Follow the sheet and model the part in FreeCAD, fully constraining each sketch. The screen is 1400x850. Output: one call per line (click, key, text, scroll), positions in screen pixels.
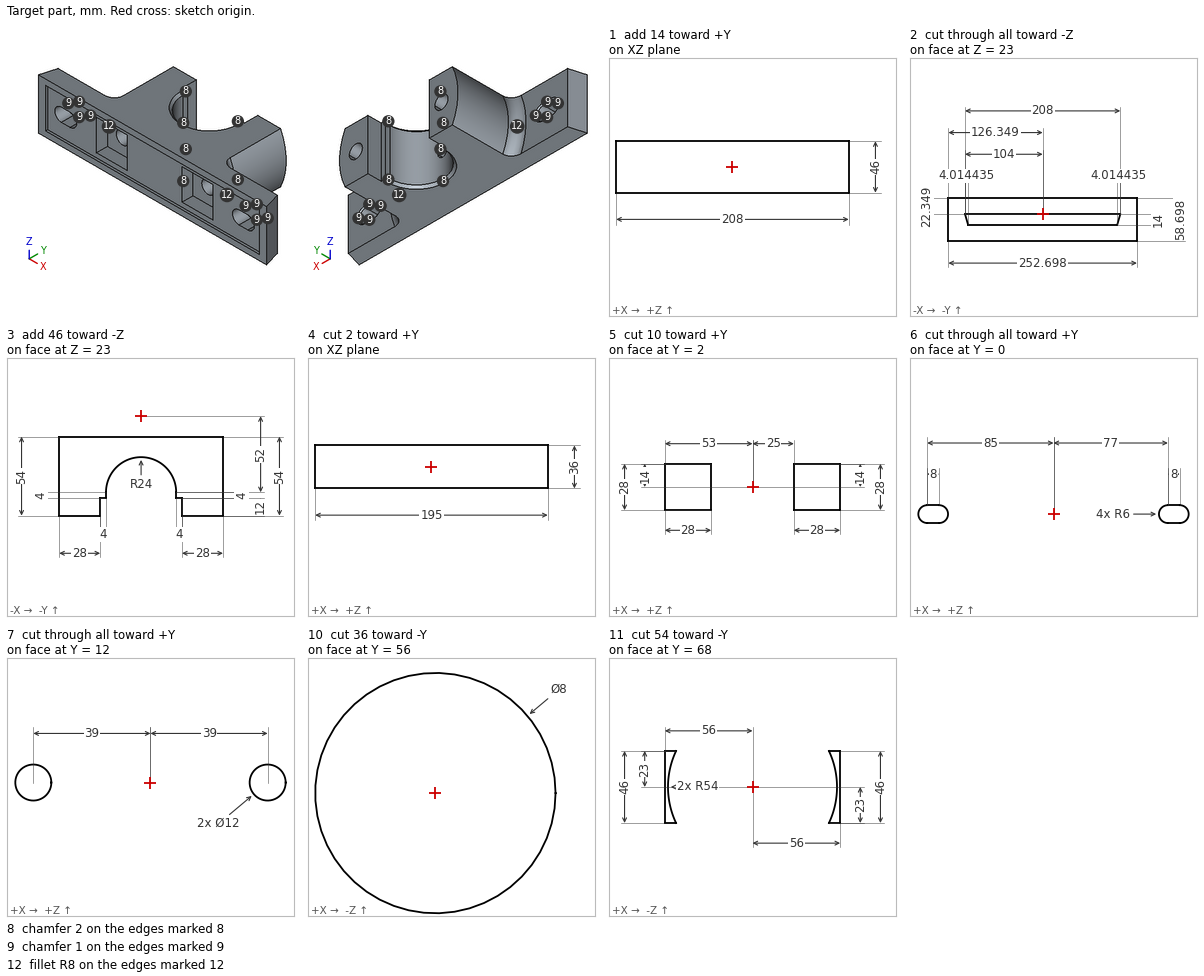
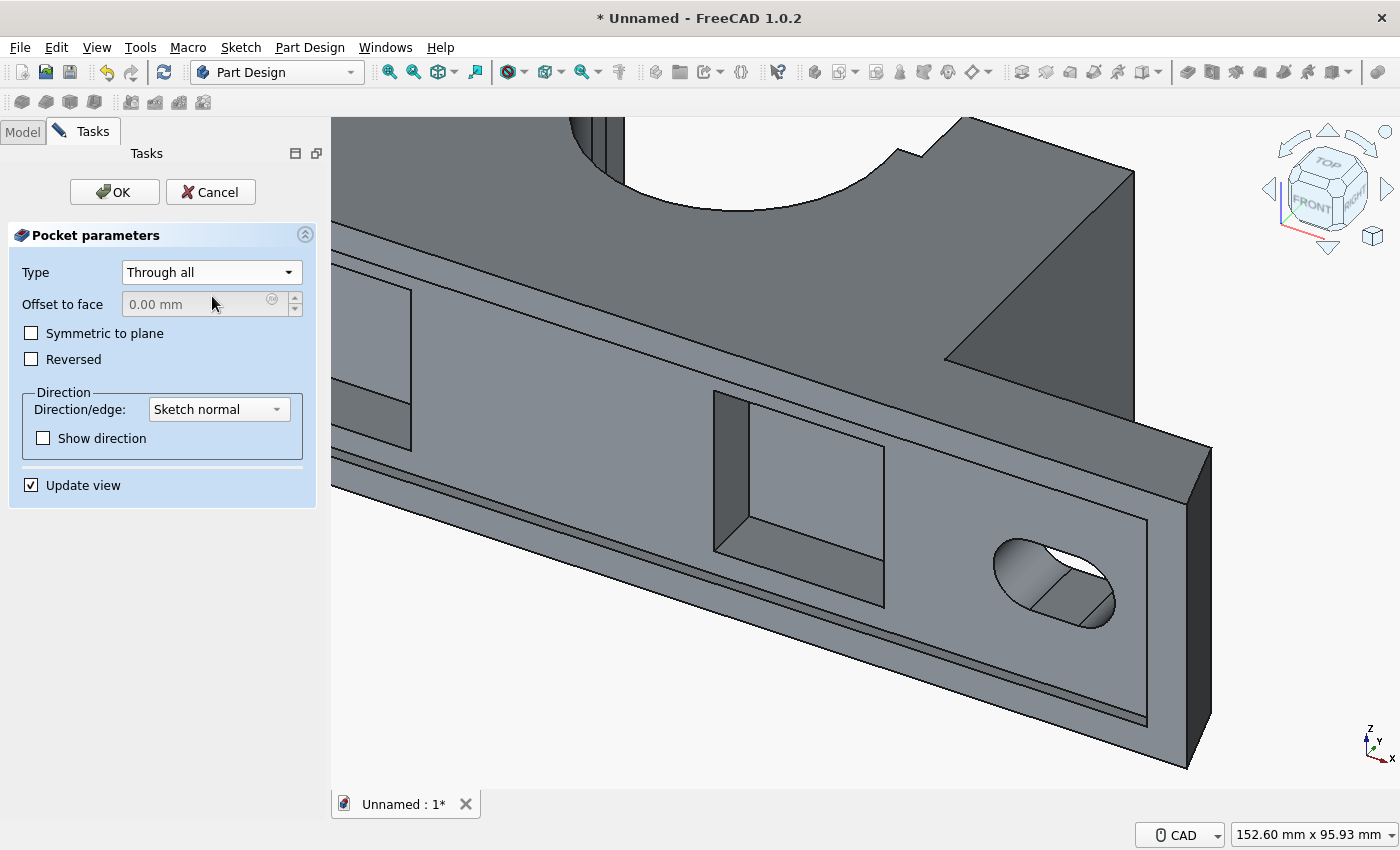
click(115, 192)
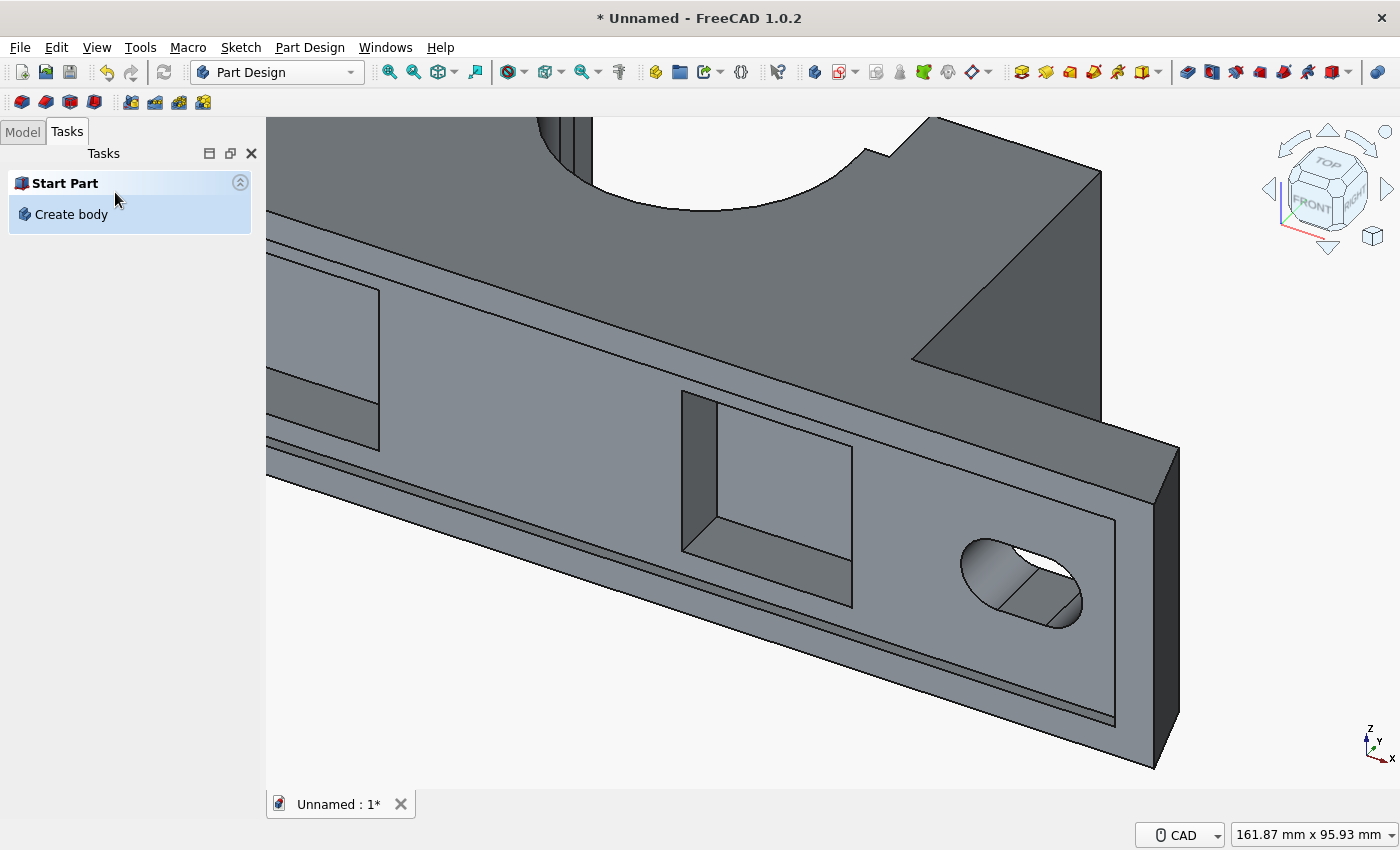
click(390, 72)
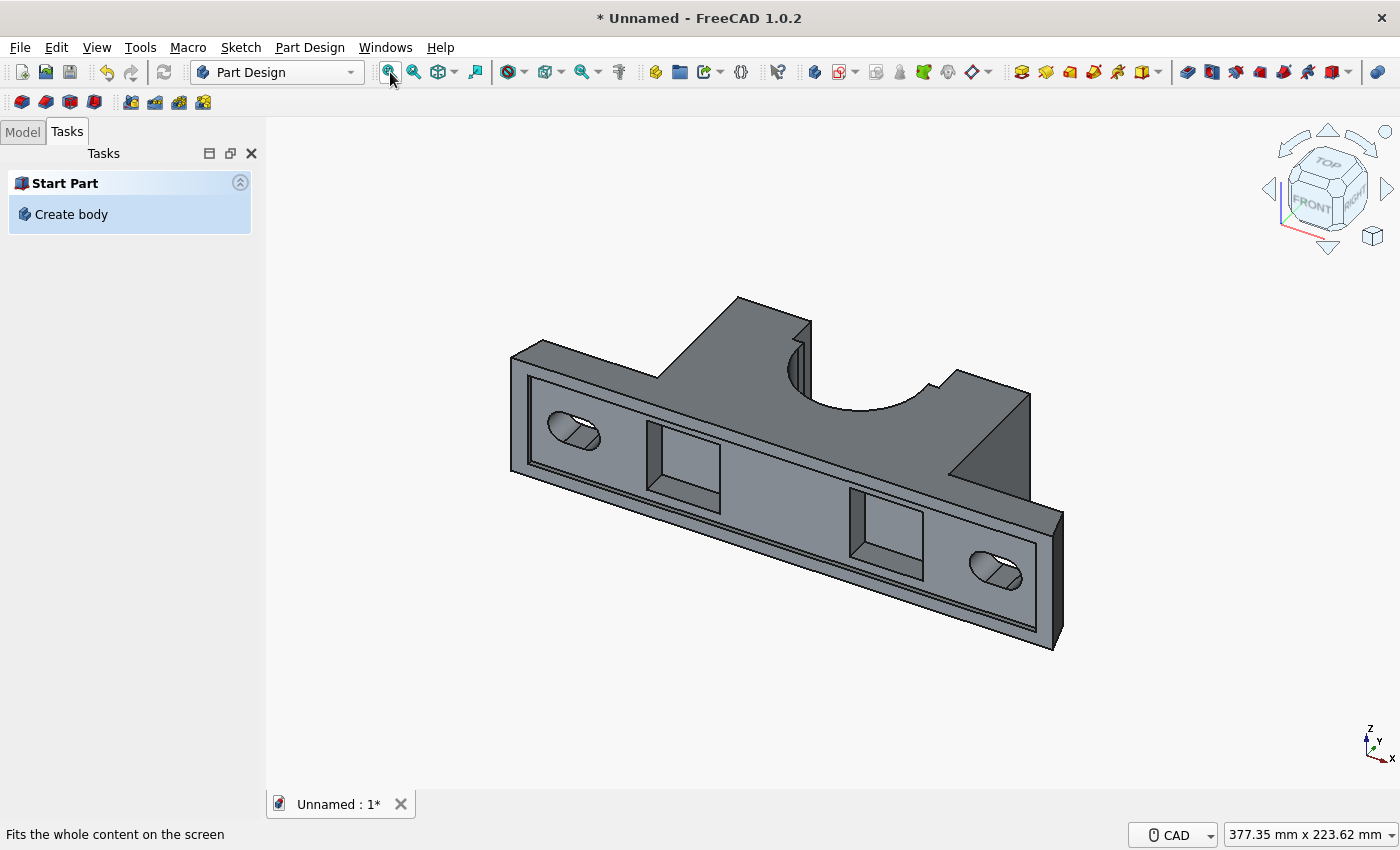
click(901, 518)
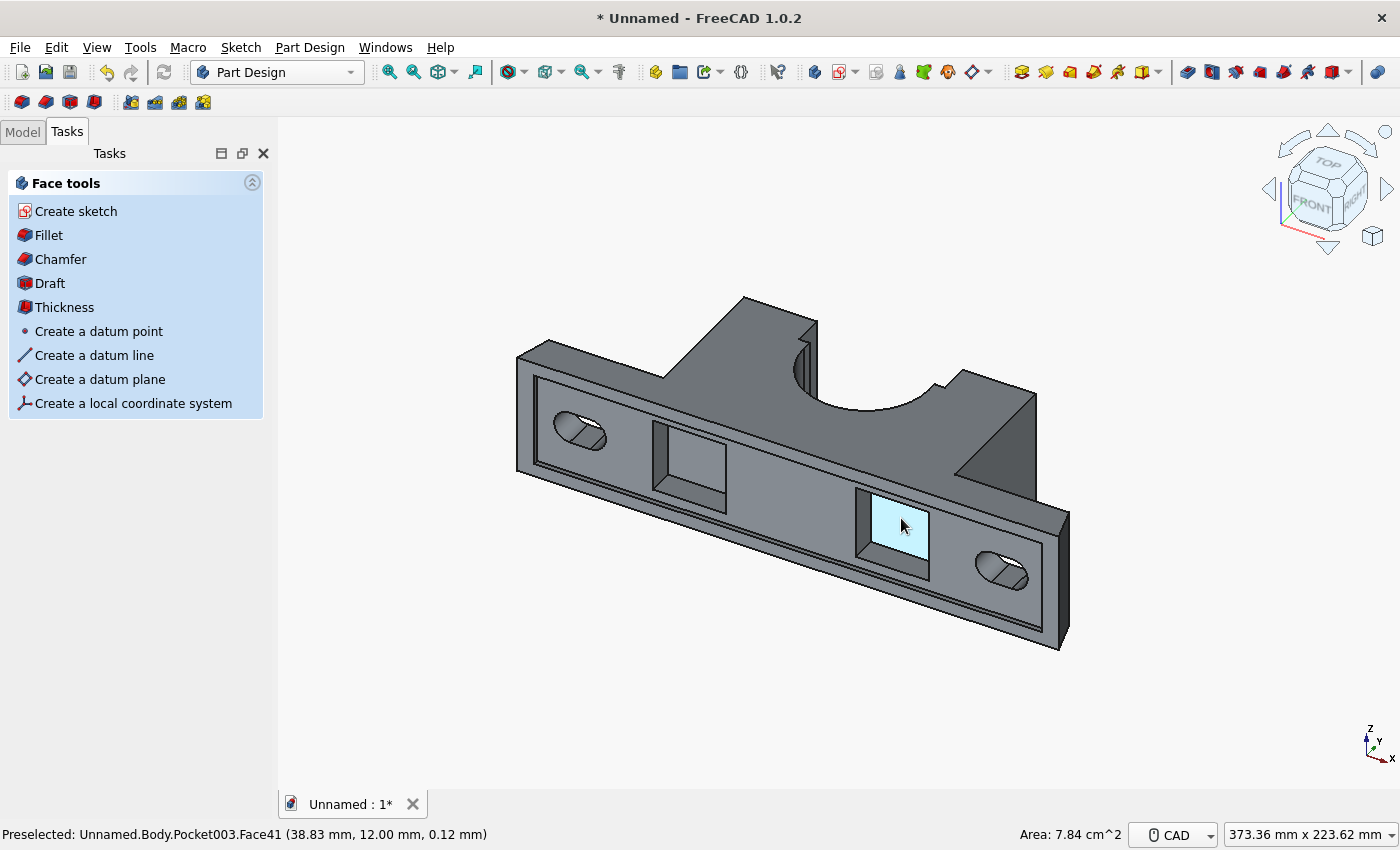
click(840, 72)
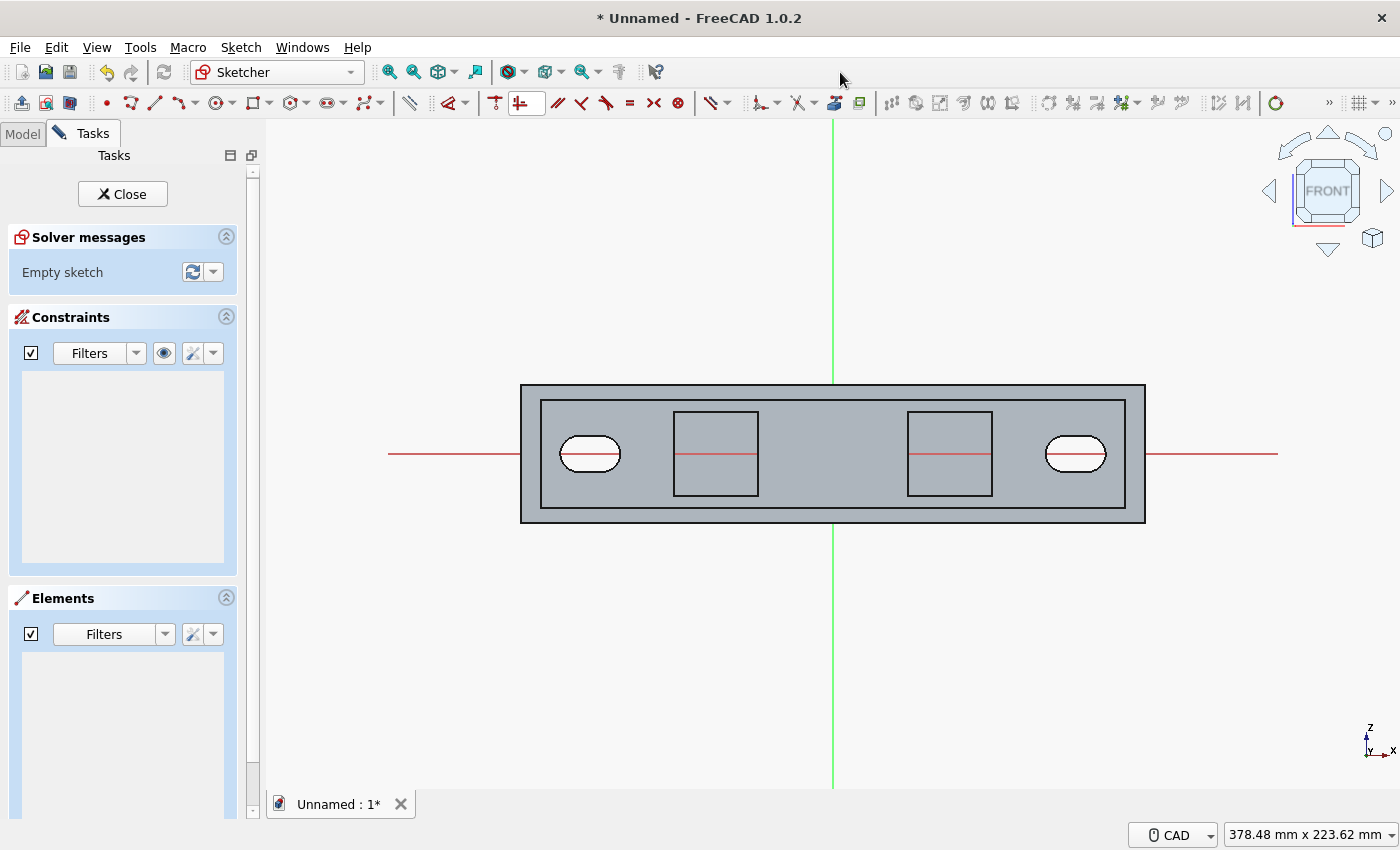
scroll(873, 454, up, 5)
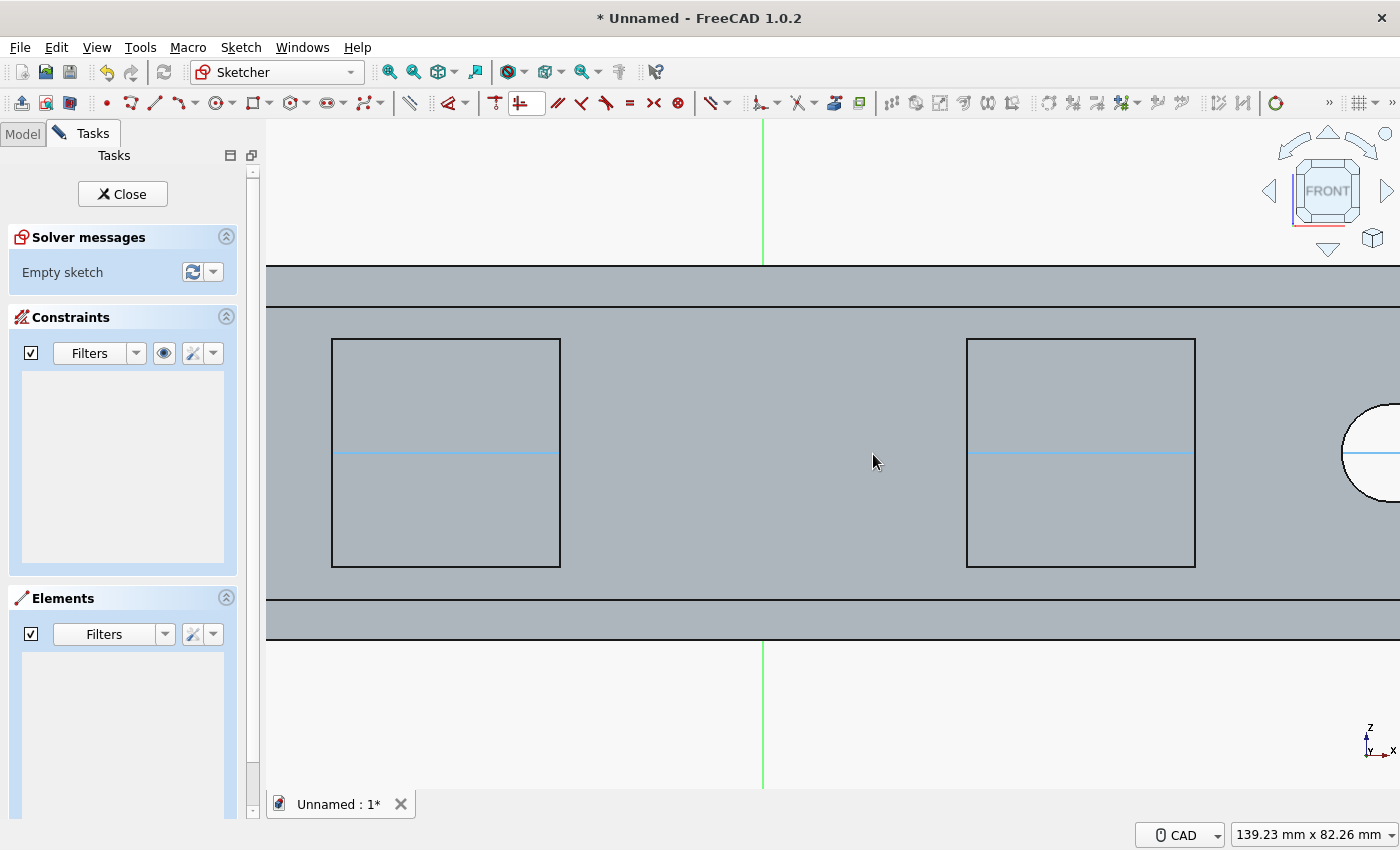
click(216, 104)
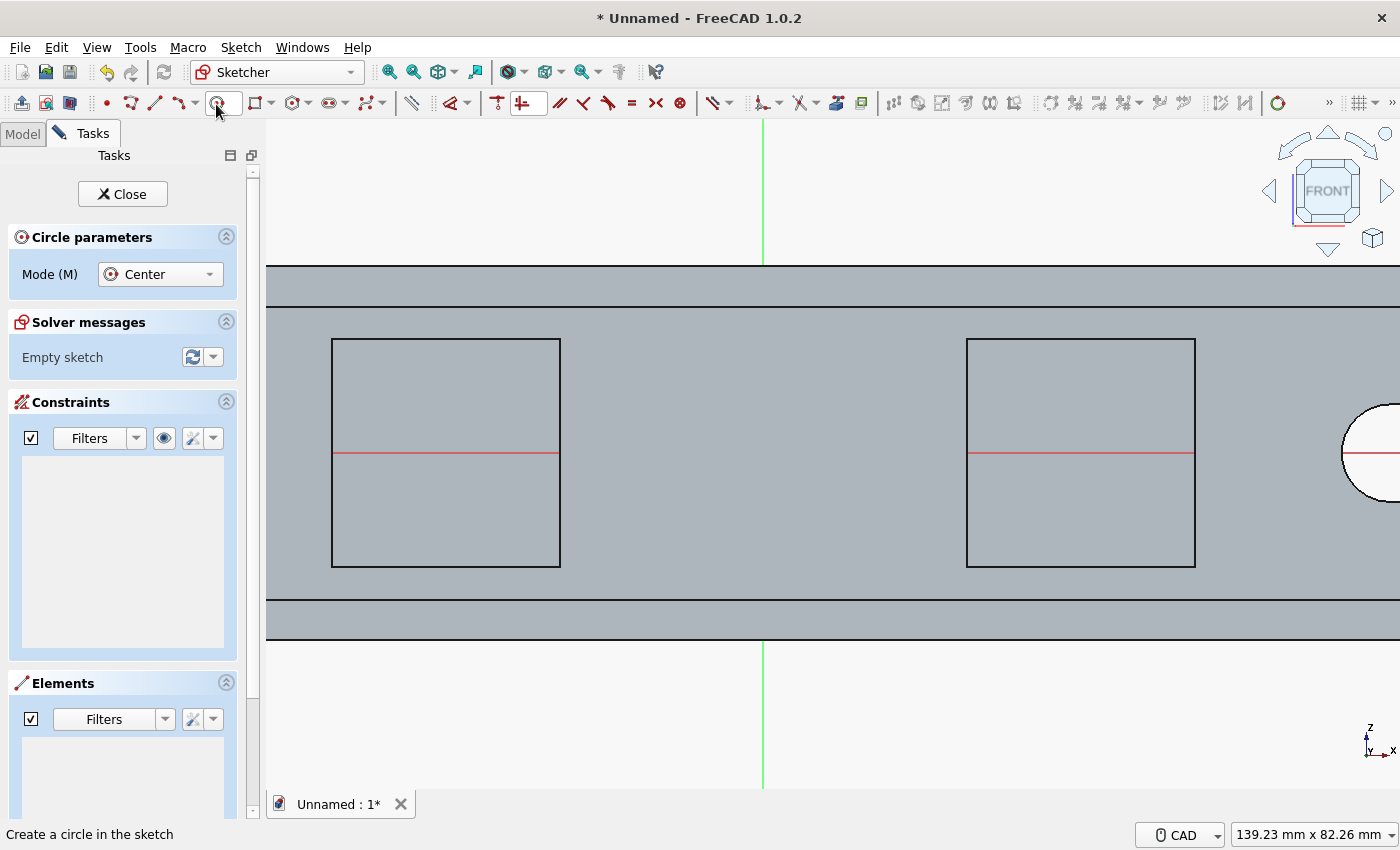
click(1081, 453)
move(1116, 419)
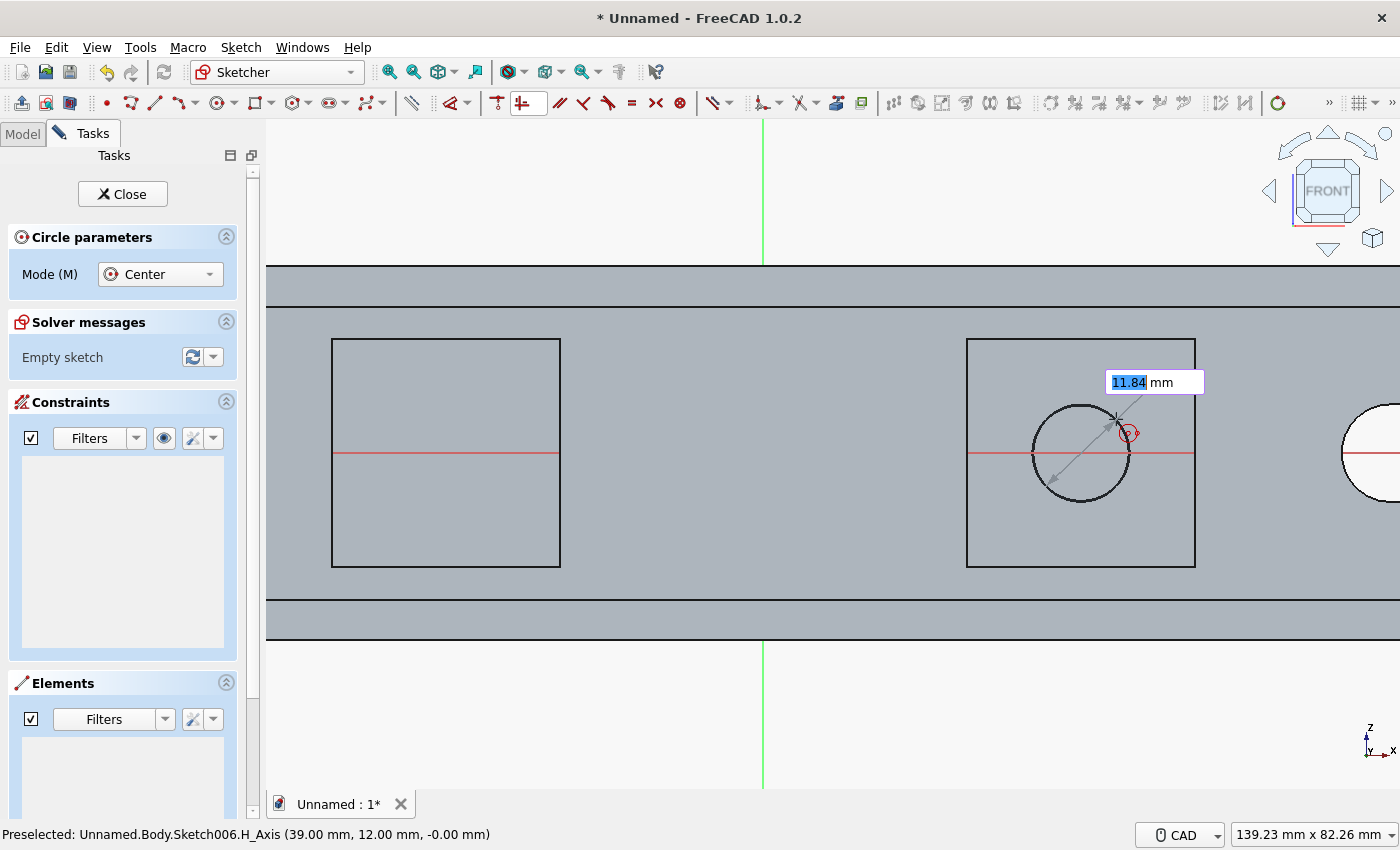
text(12)
key(Return)